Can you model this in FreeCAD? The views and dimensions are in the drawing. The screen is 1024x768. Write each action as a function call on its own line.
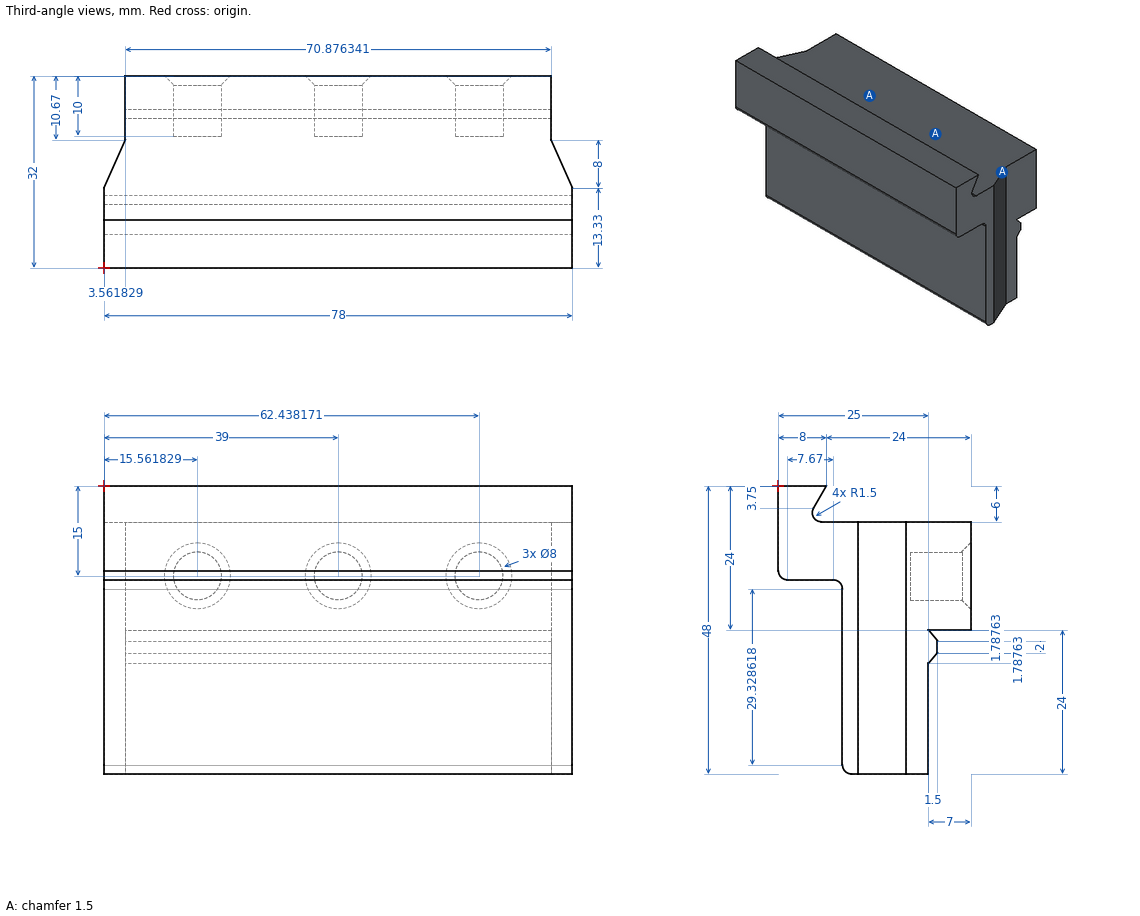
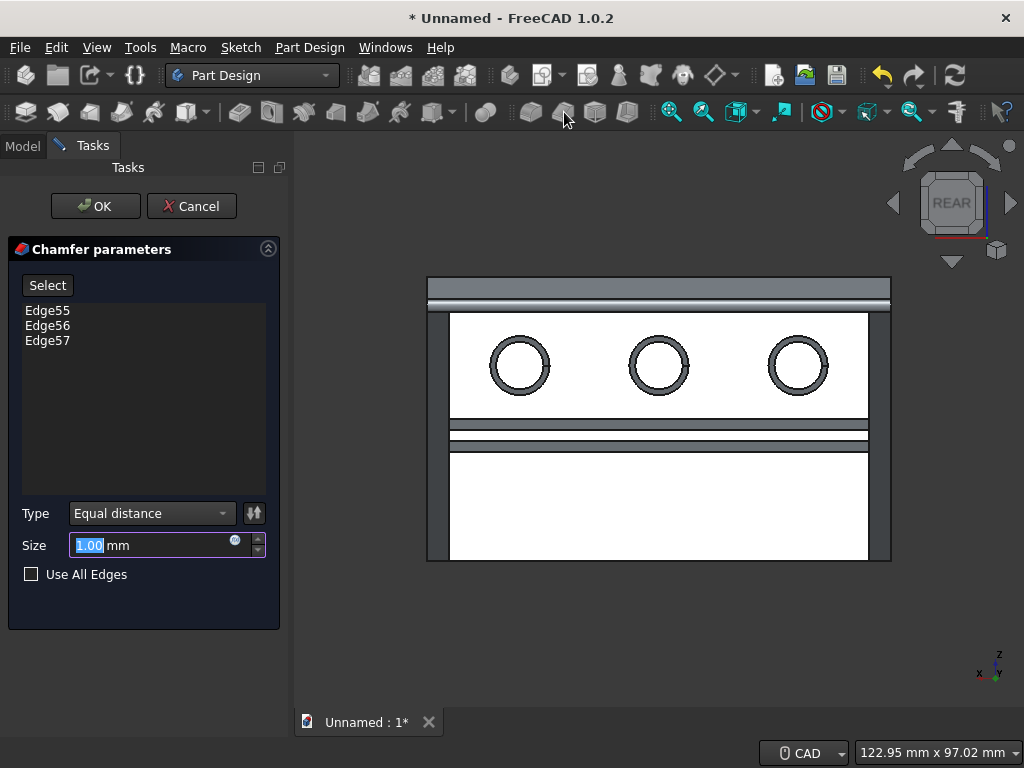
text(1.5)
key(Tab)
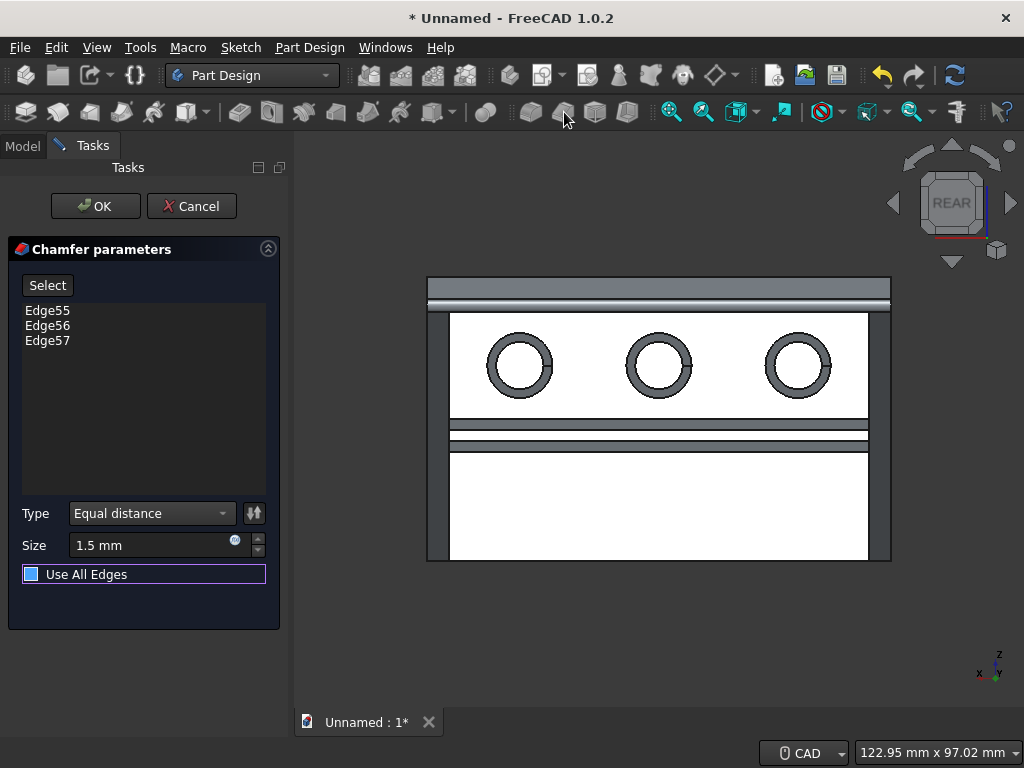
click(96, 206)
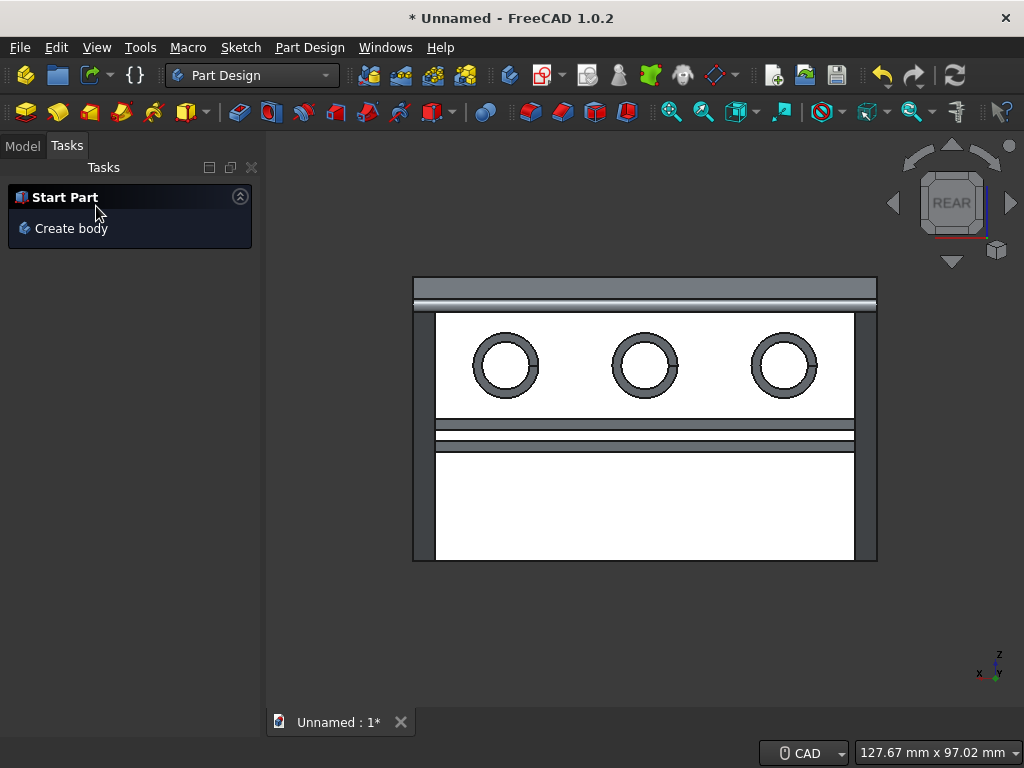
key(0)